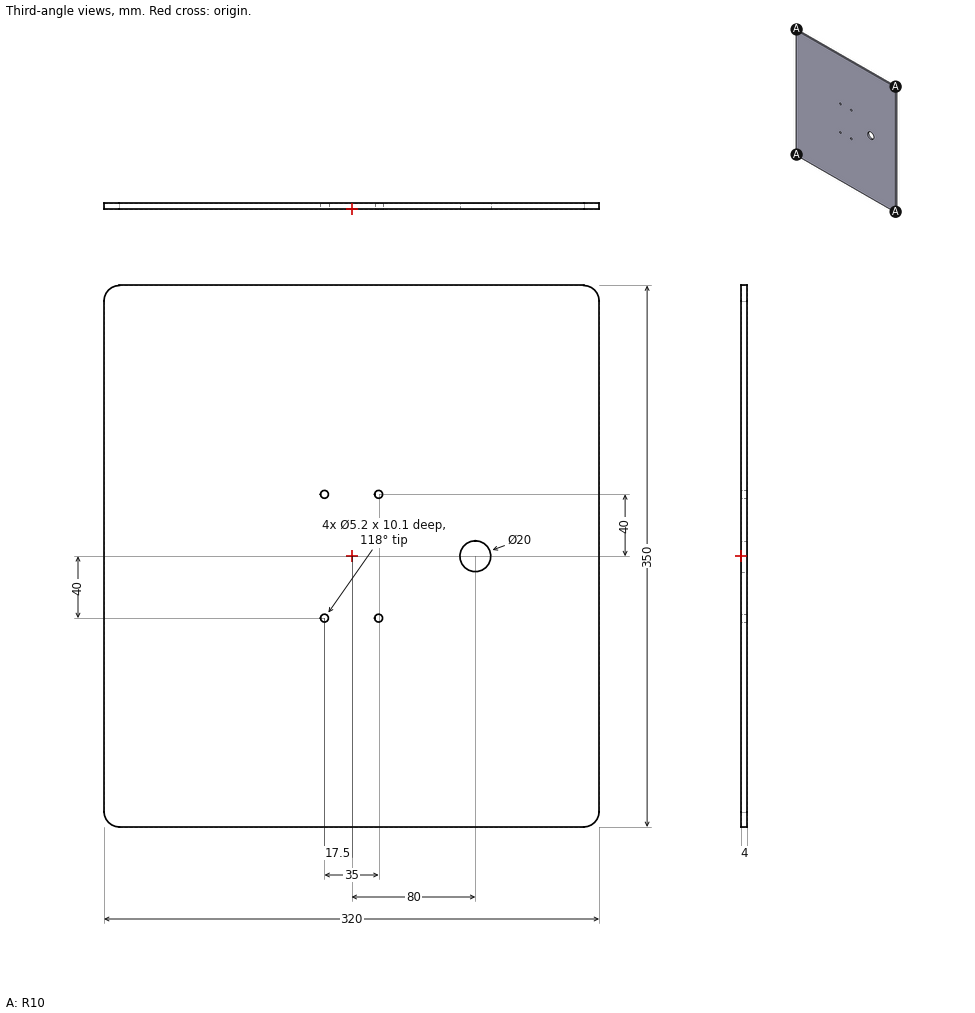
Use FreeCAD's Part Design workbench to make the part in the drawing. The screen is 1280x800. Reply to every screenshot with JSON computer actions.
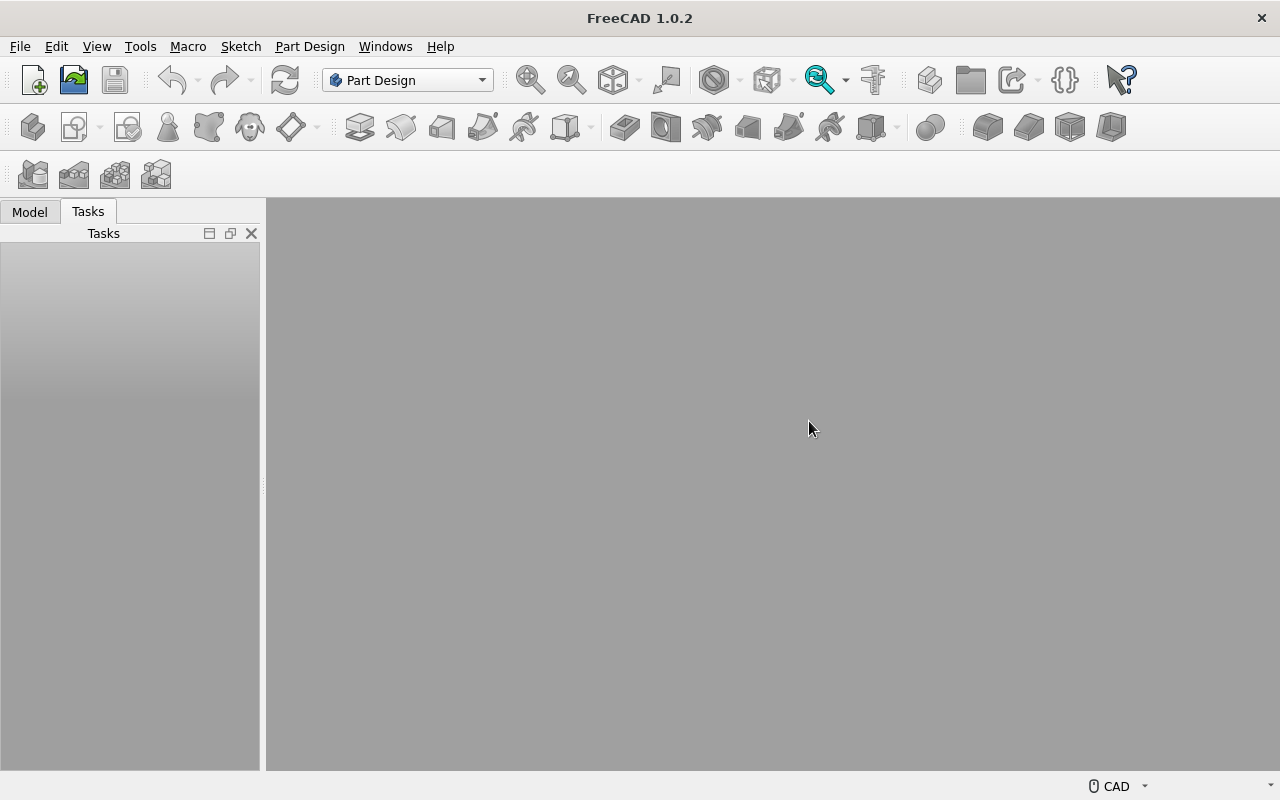
{"action": "left_click", "coordinate": [33, 80]}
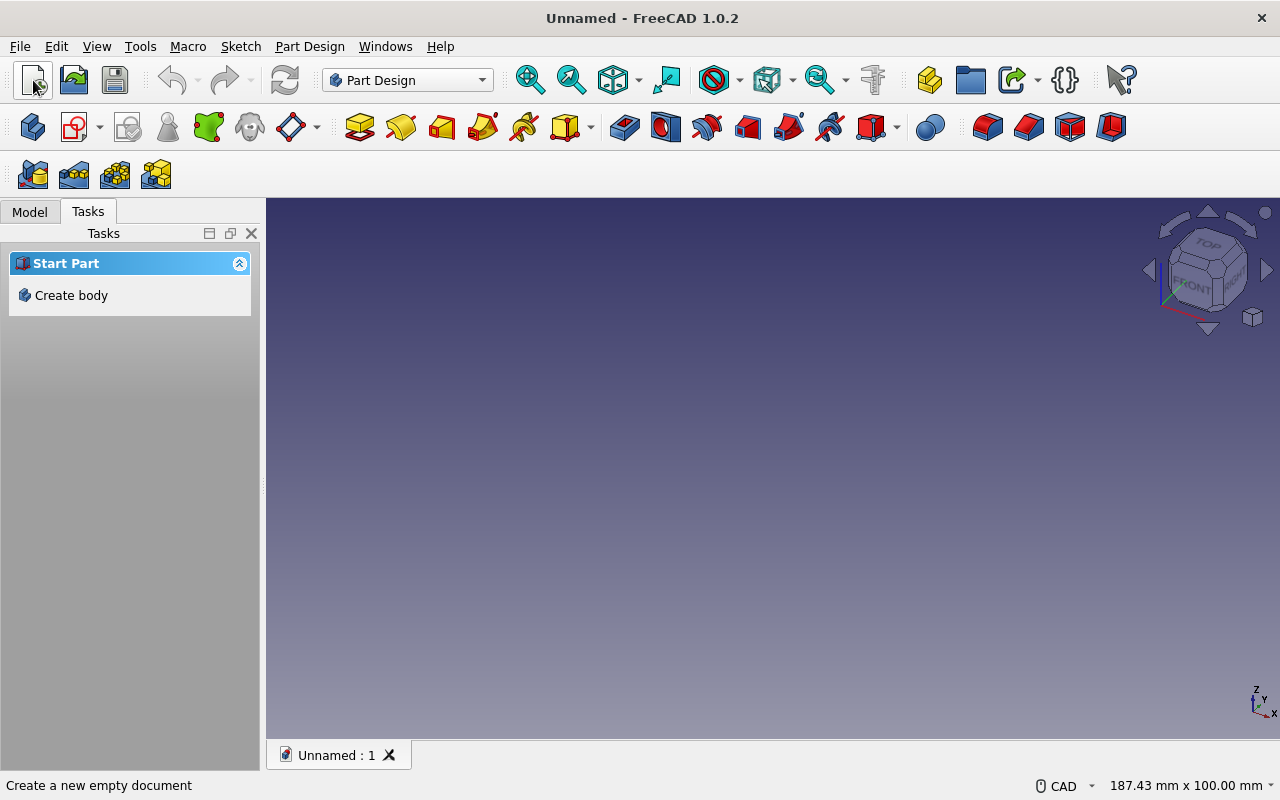
{"action": "left_click", "coordinate": [74, 128]}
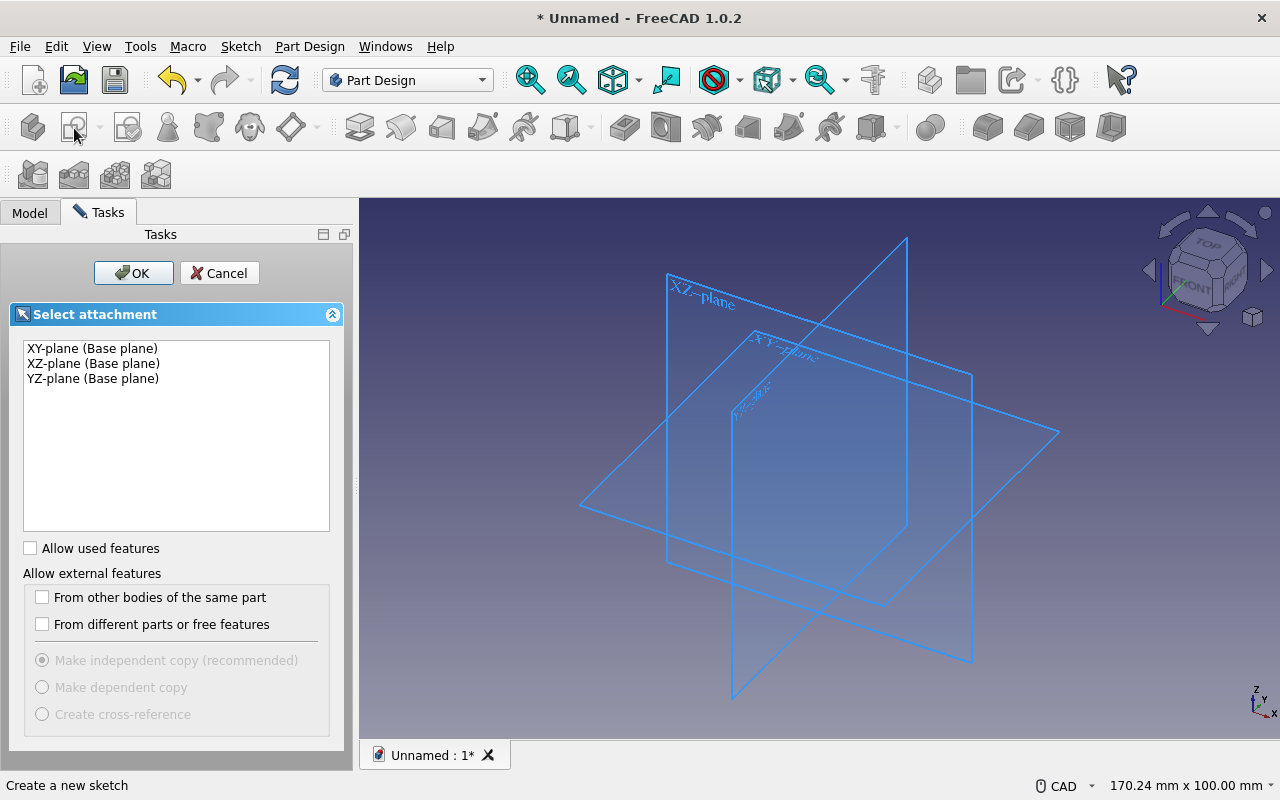
{"action": "left_click", "coordinate": [84, 364]}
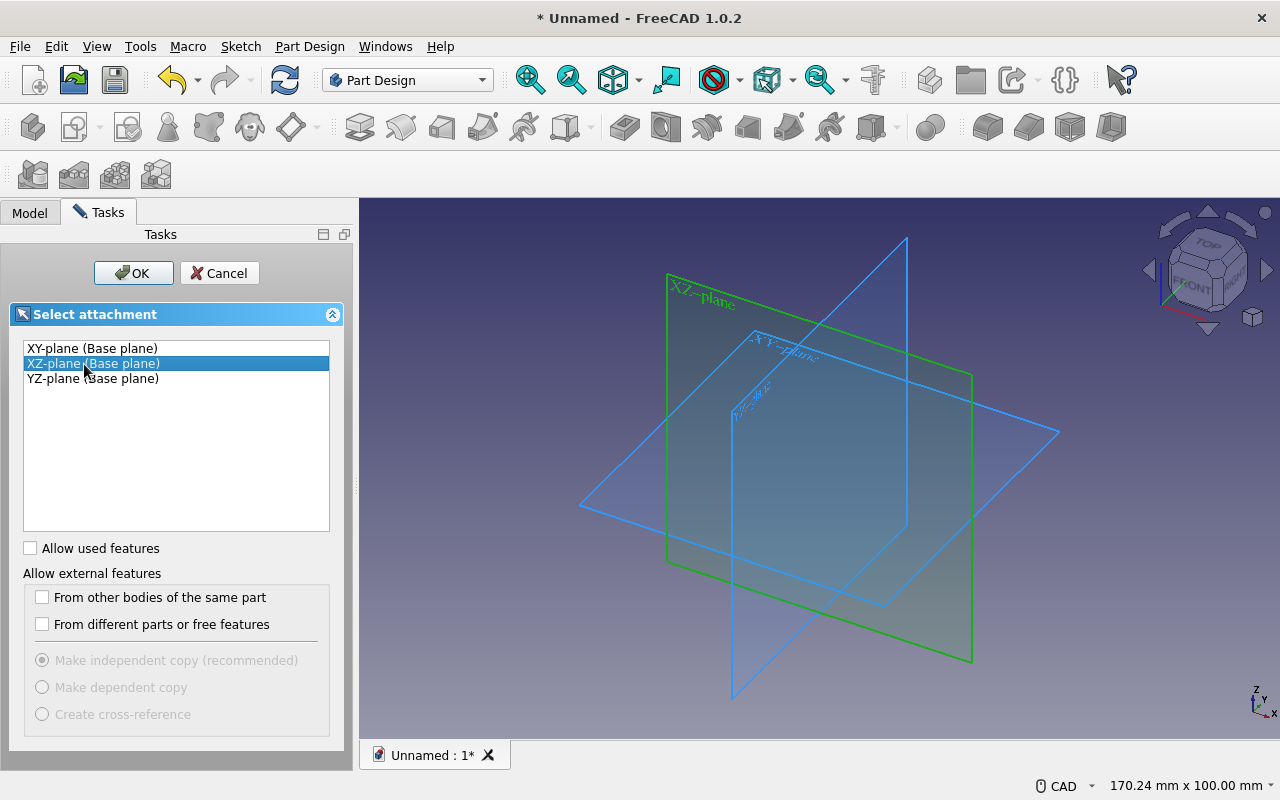
{"action": "left_click", "coordinate": [134, 273]}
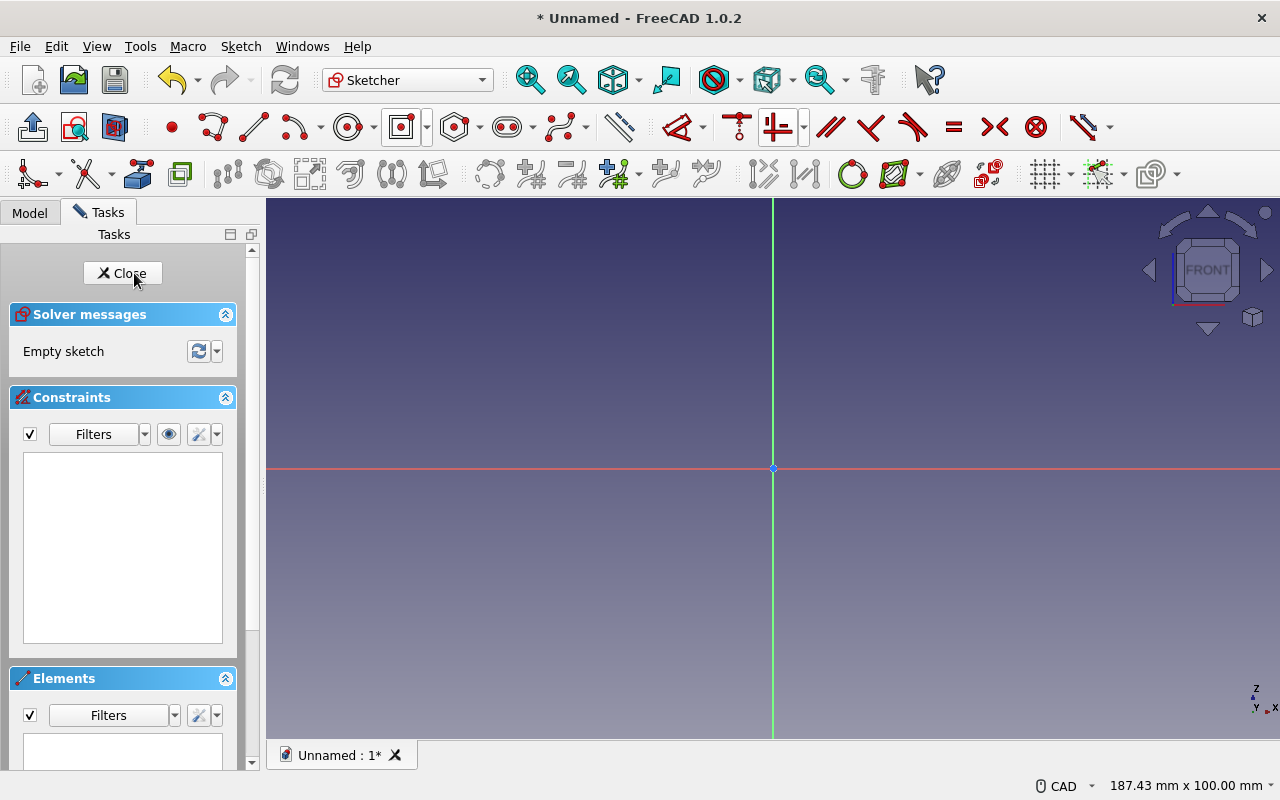
{"action": "scroll", "coordinate": [691, 468], "scroll_direction": "down", "scroll_amount": 9}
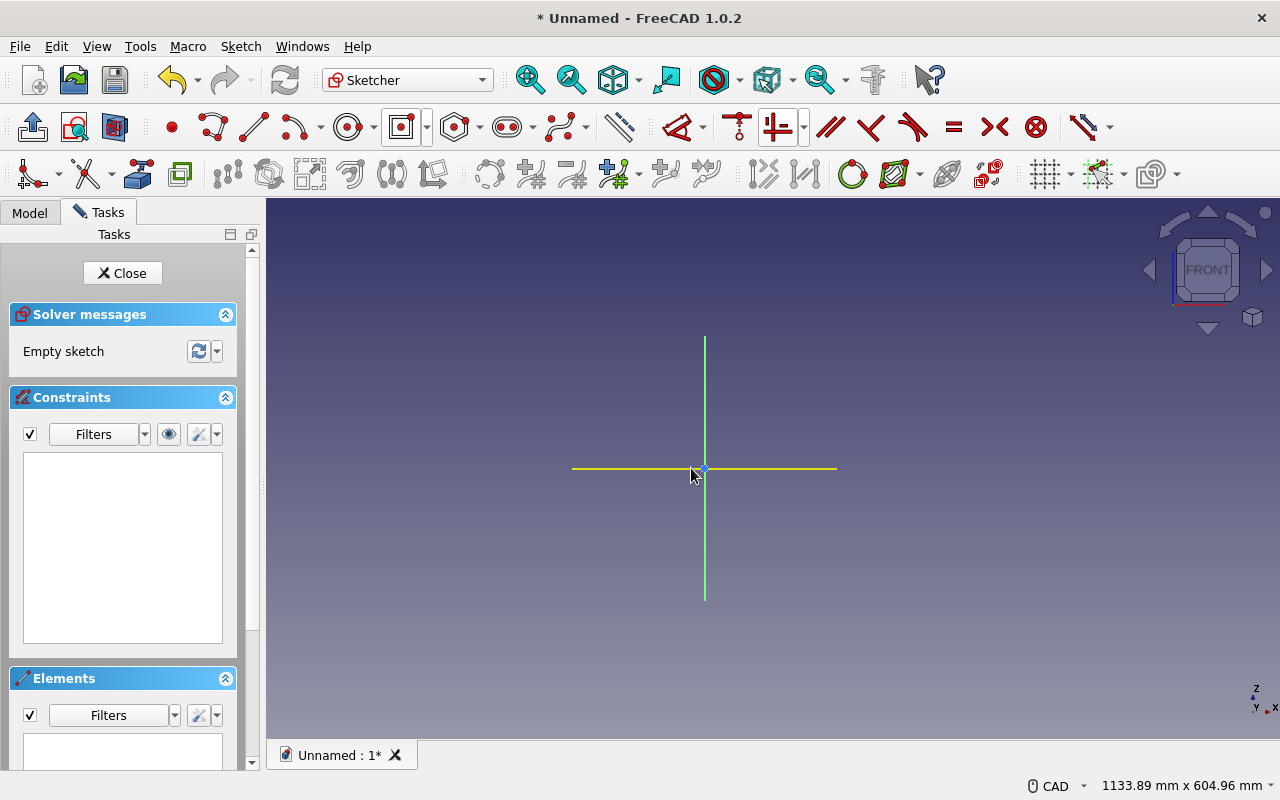
{"action": "left_click", "coordinate": [400, 128]}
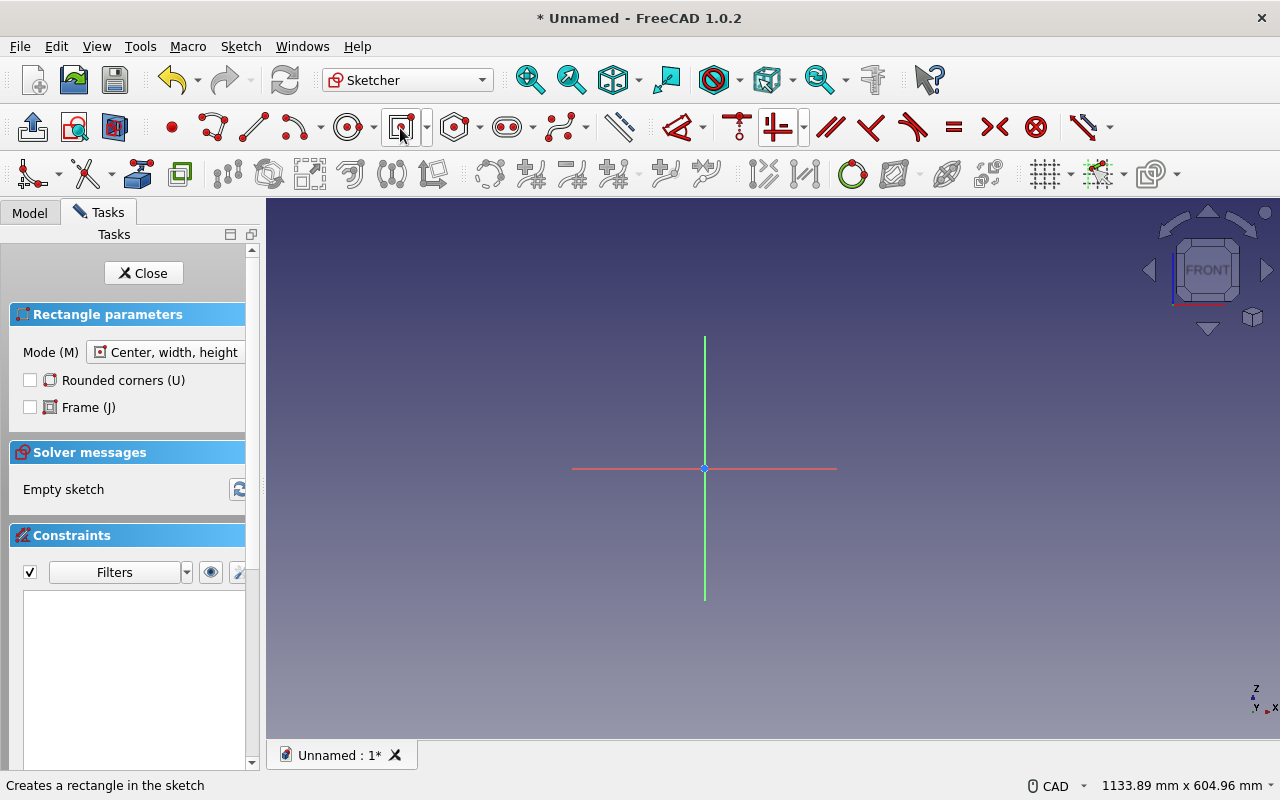
{"action": "left_click", "coordinate": [705, 468]}
{"action": "left_click", "coordinate": [848, 312]}
{"action": "key", "text": "Escape"}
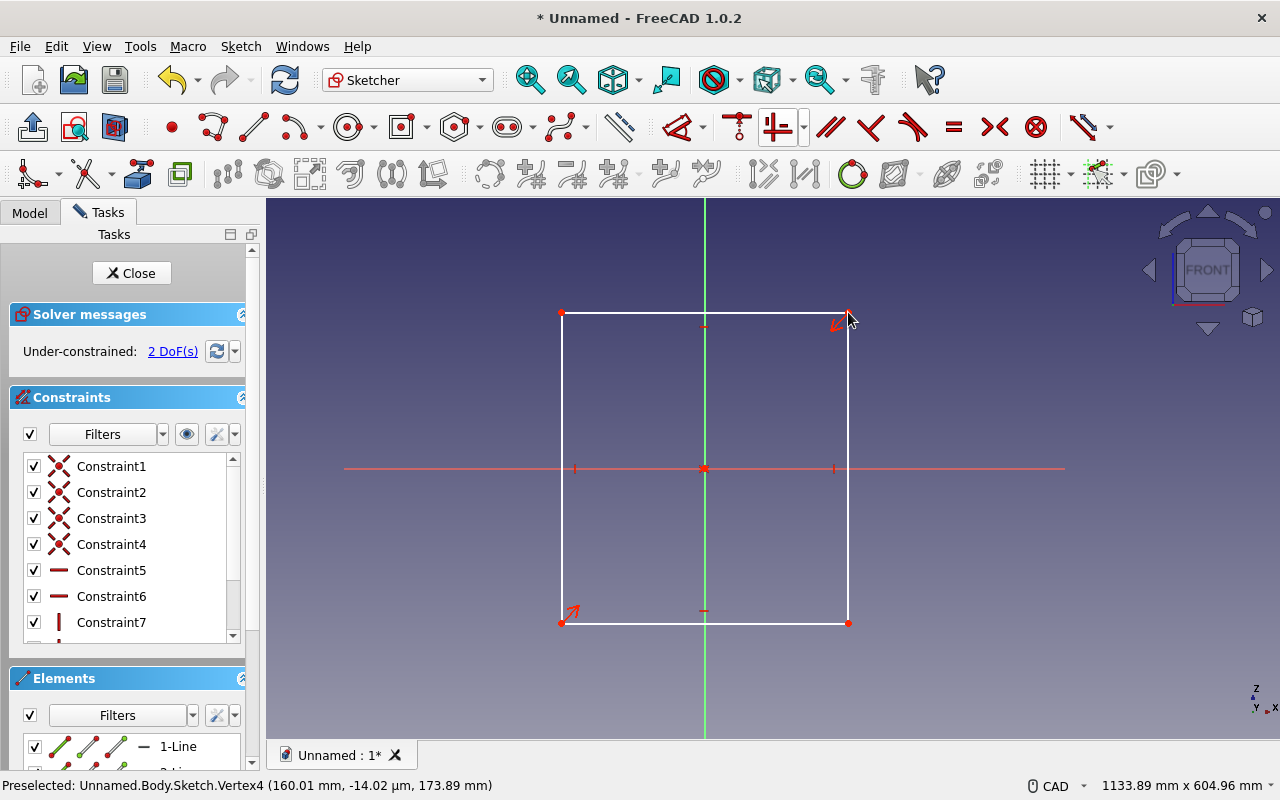
{"action": "left_click", "coordinate": [676, 128]}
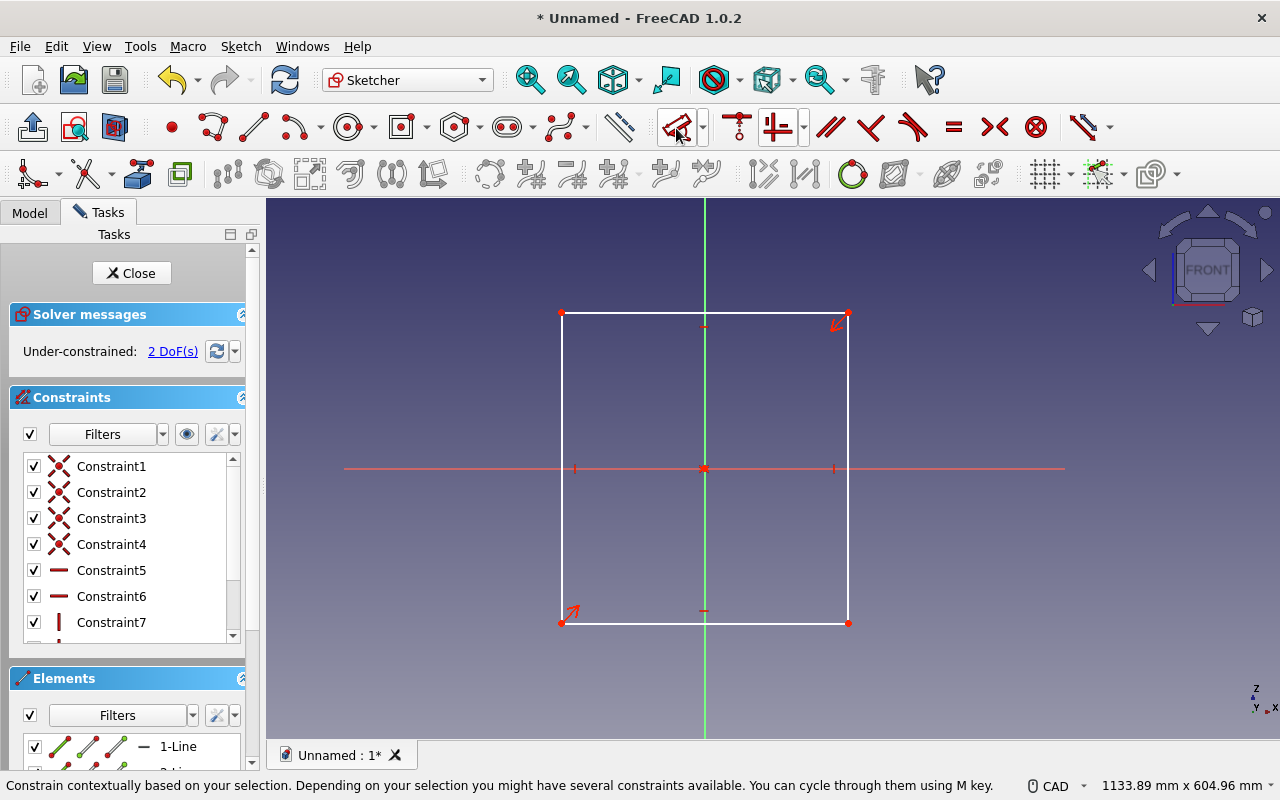
{"action": "left_click", "coordinate": [648, 624]}
{"action": "left_click", "coordinate": [639, 658]}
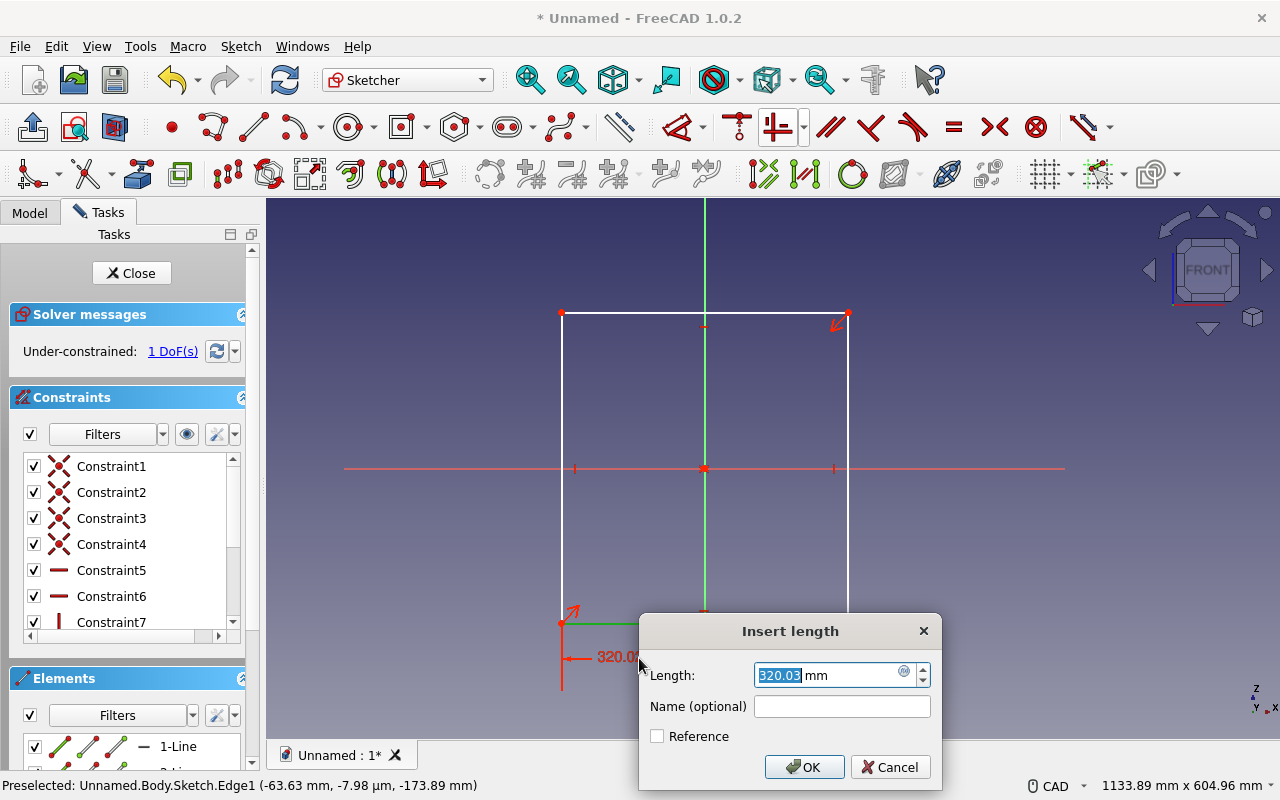
{"action": "type", "text": "320"}
{"action": "key", "text": "Return"}